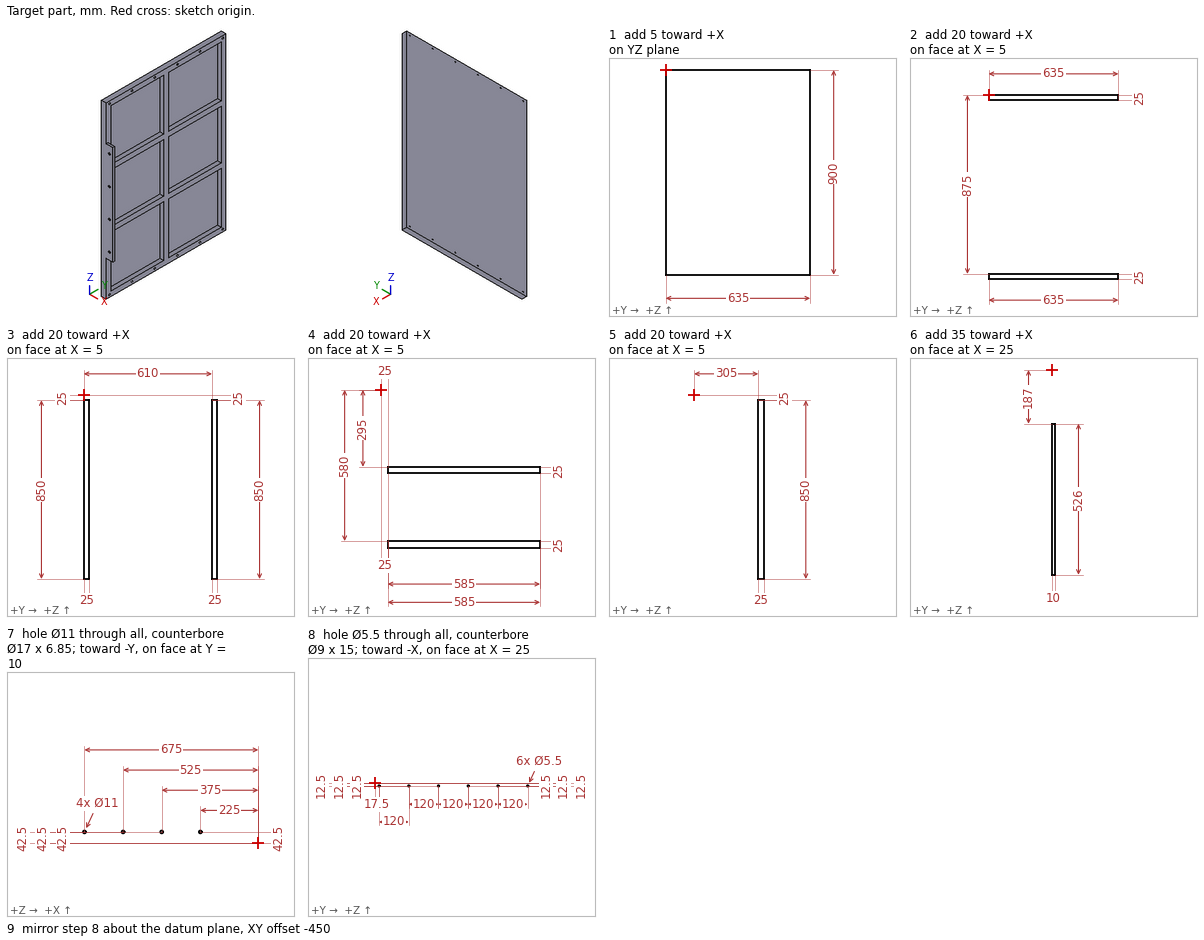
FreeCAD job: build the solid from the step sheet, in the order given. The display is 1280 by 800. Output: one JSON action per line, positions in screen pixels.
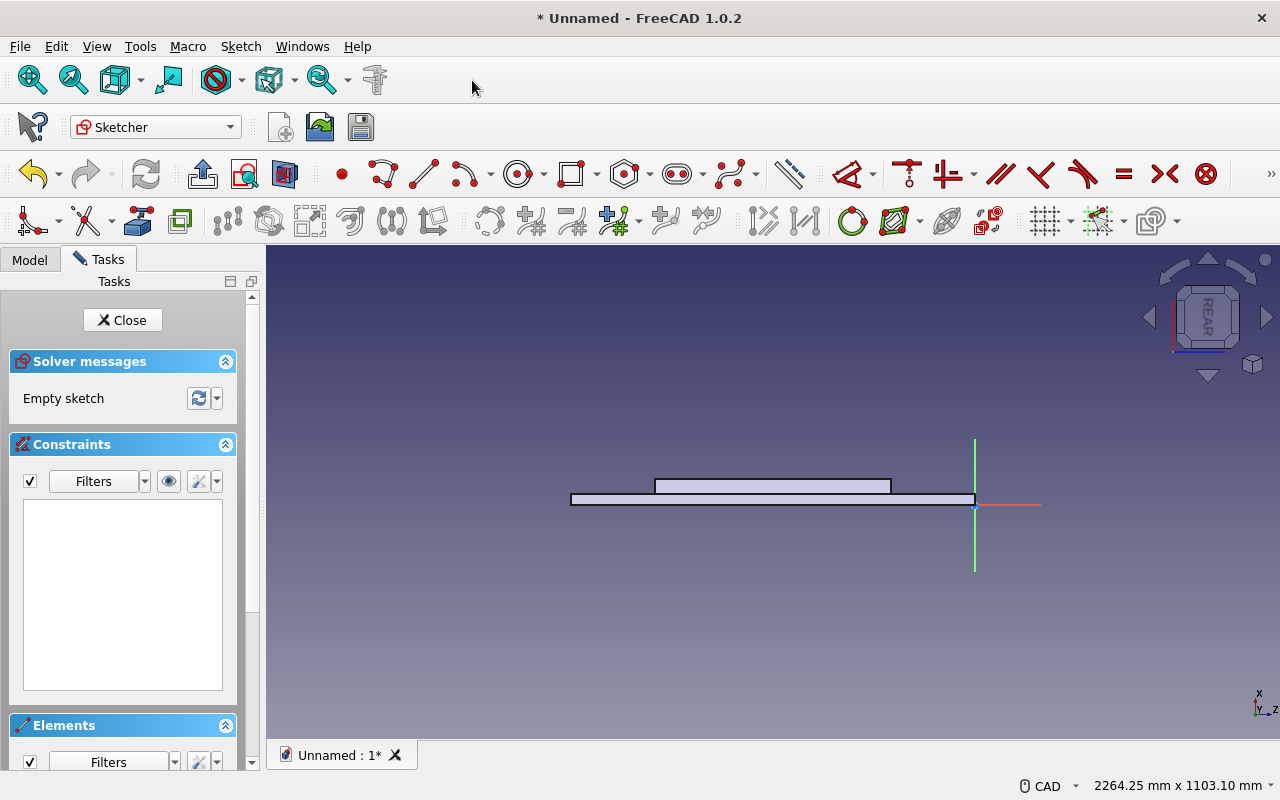
{"action": "scroll", "coordinate": [965, 498], "scroll_direction": "up", "scroll_amount": 3}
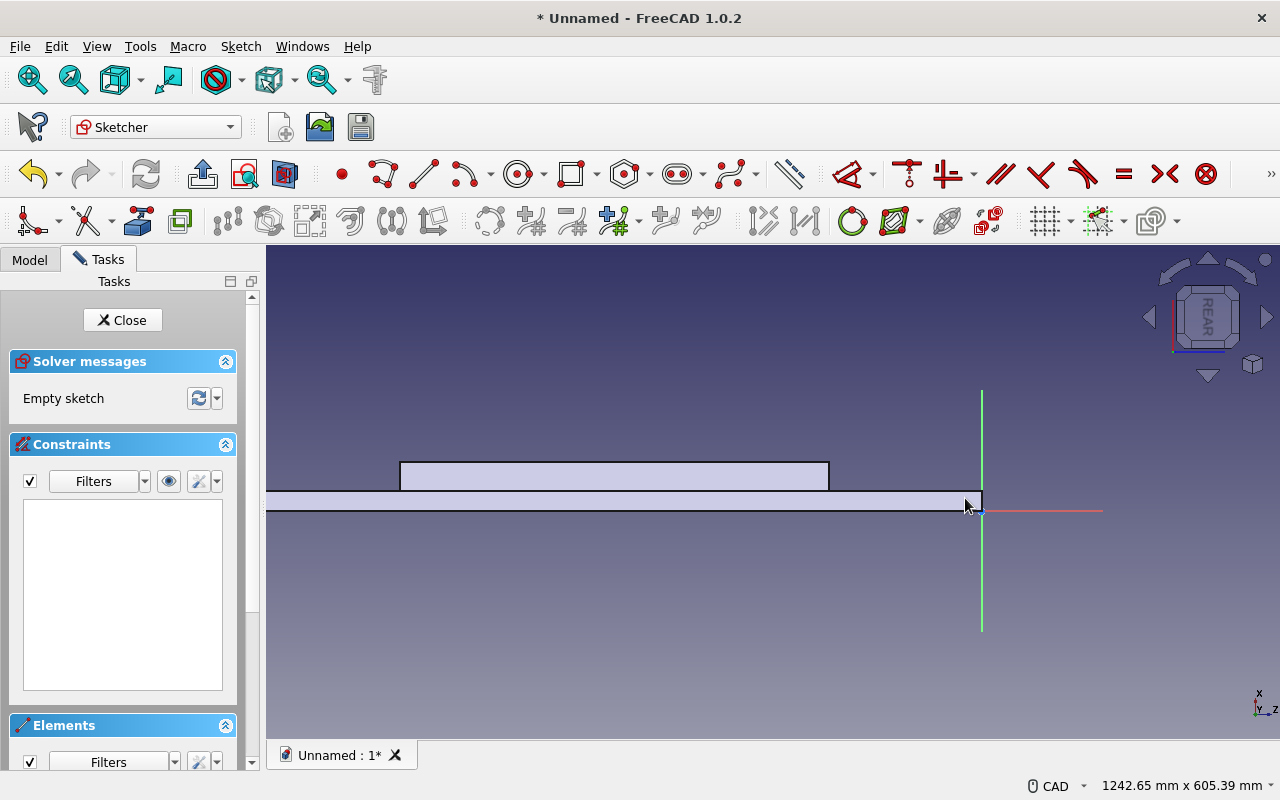
{"action": "left_click", "coordinate": [518, 174]}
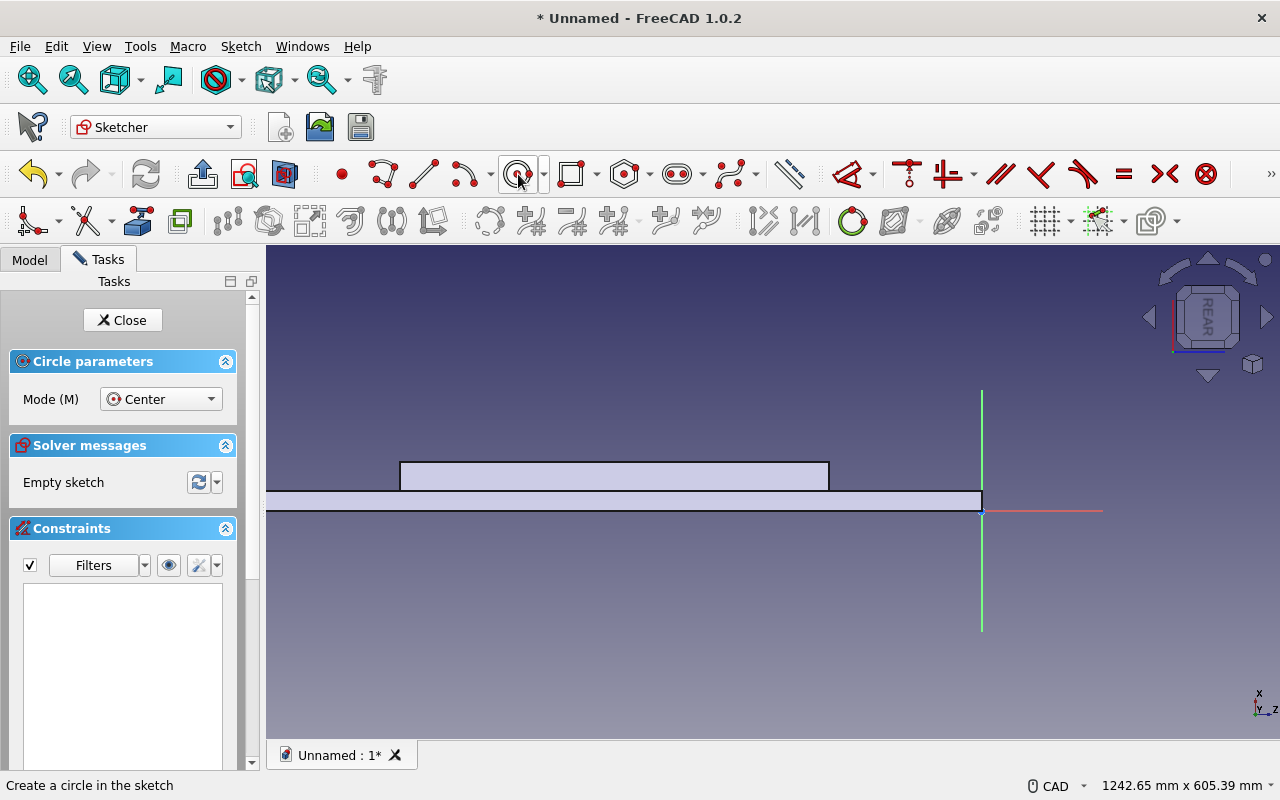
{"action": "scroll", "coordinate": [431, 476], "scroll_direction": "up", "scroll_amount": 9}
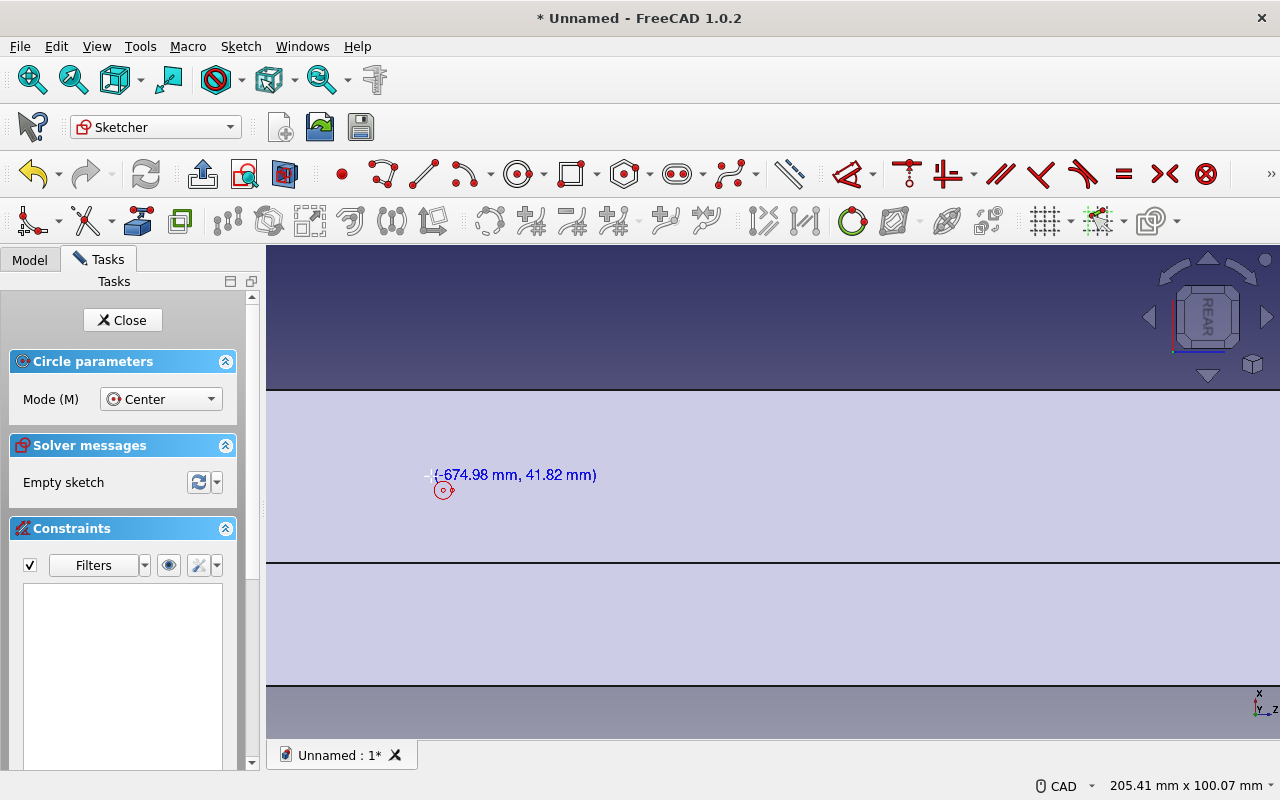
{"action": "scroll", "coordinate": [432, 477], "scroll_direction": "down", "scroll_amount": 9}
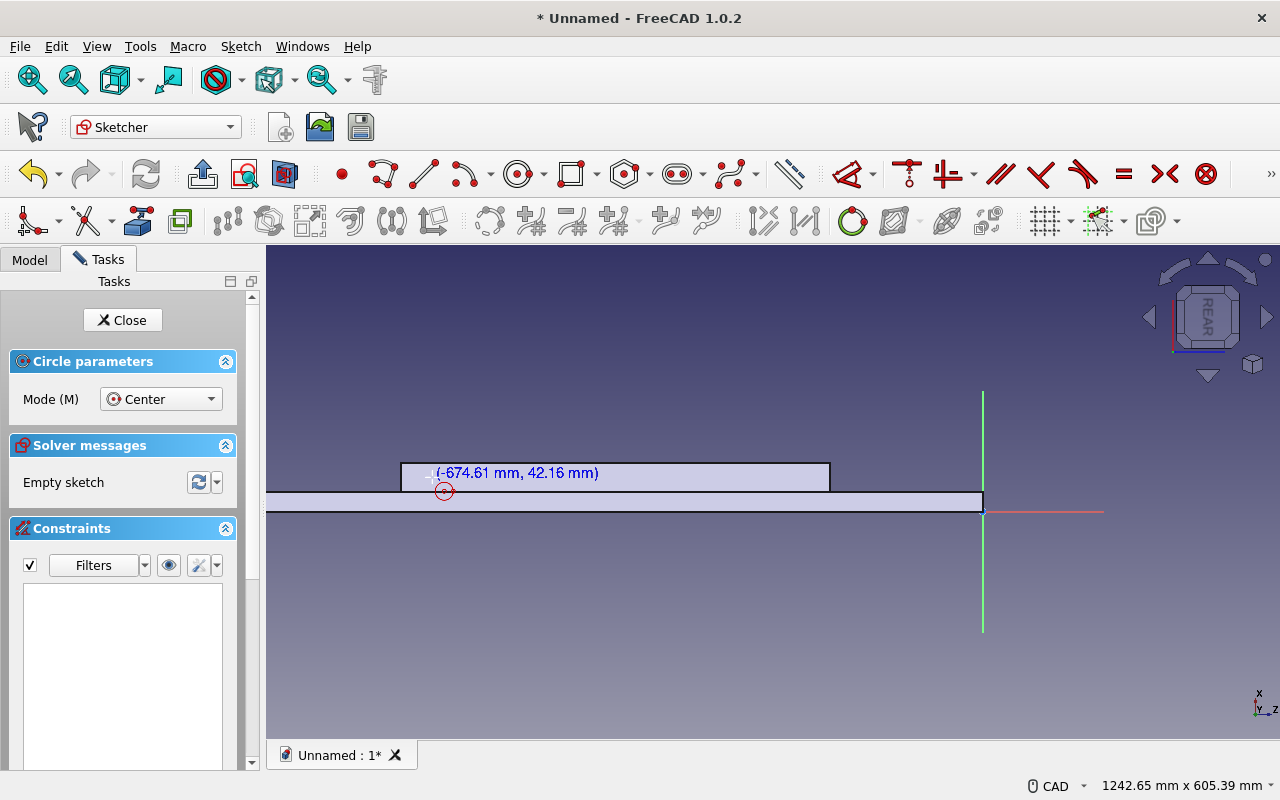
{"action": "left_click", "coordinate": [432, 477]}
{"action": "mouse_move", "coordinate": [435, 474]}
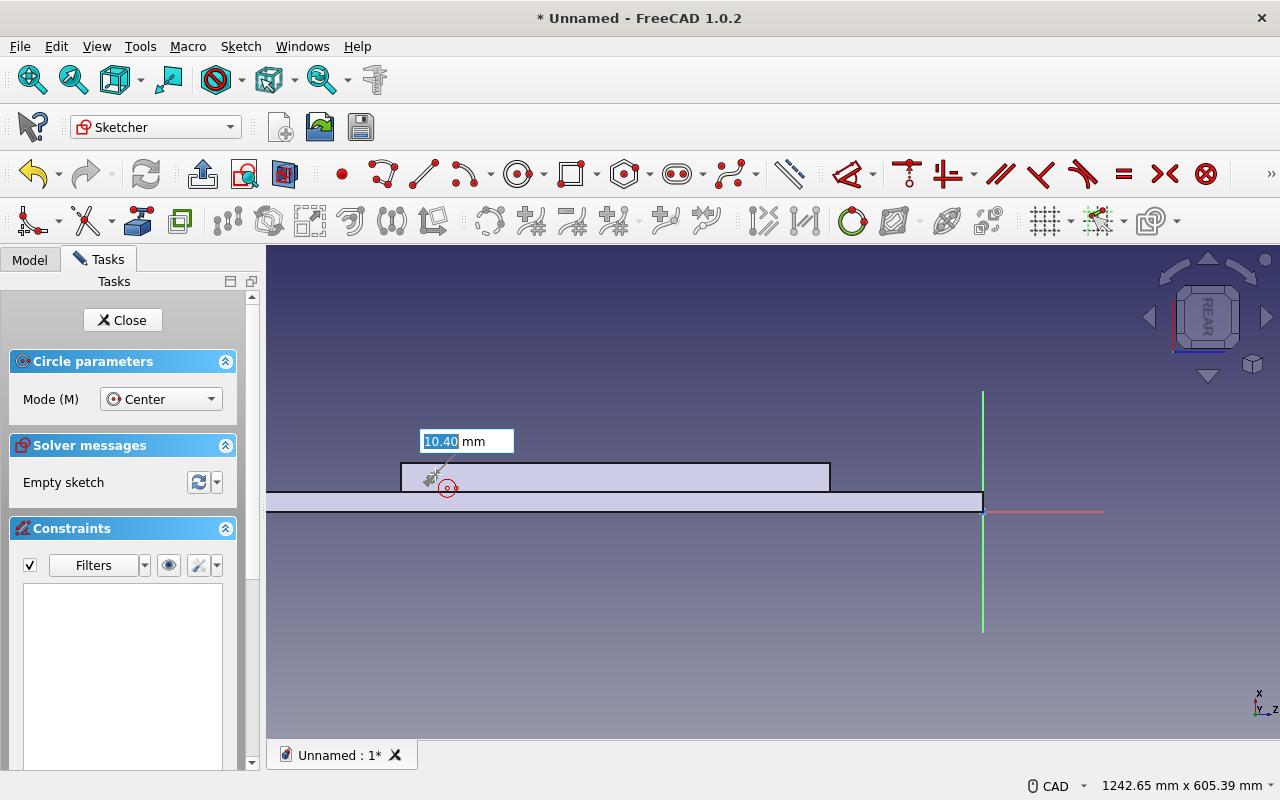
{"action": "type", "text": "11"}
{"action": "key", "text": "Return"}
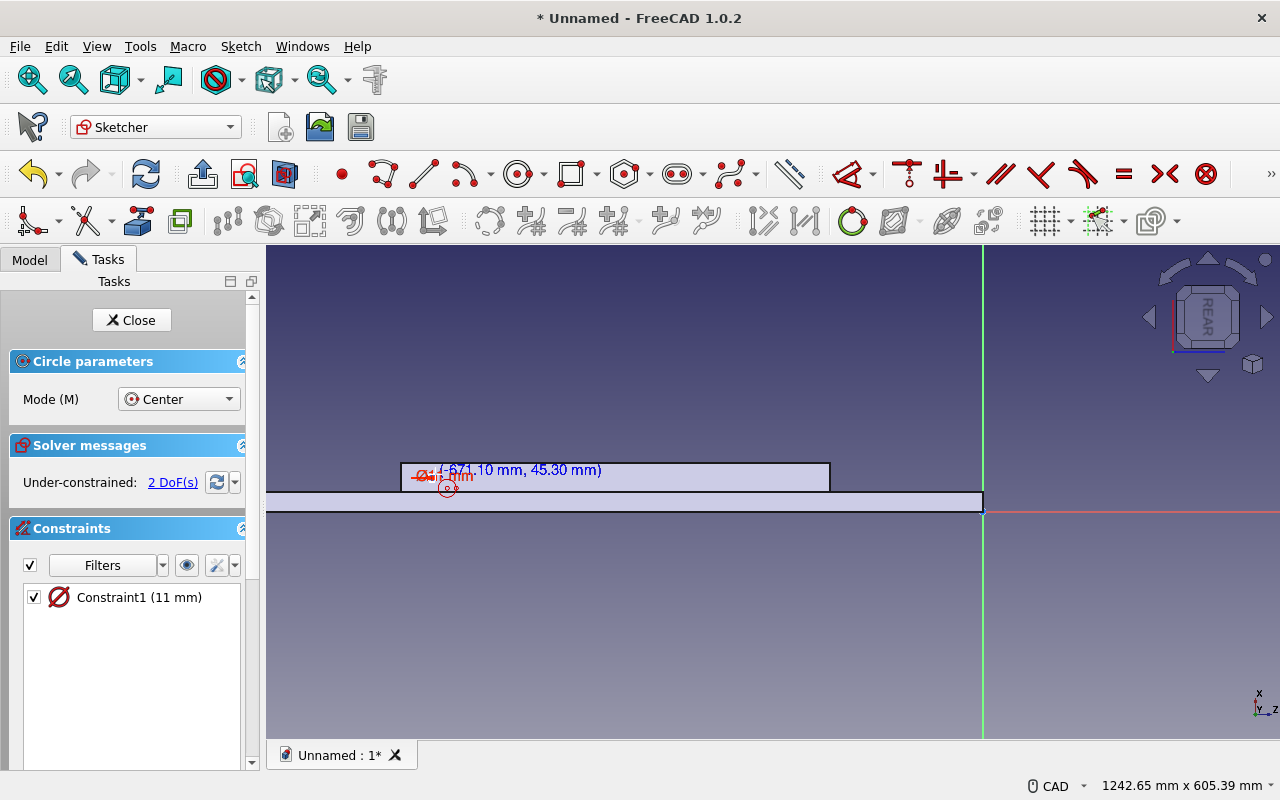
{"action": "scroll", "coordinate": [554, 477], "scroll_direction": "up", "scroll_amount": 9}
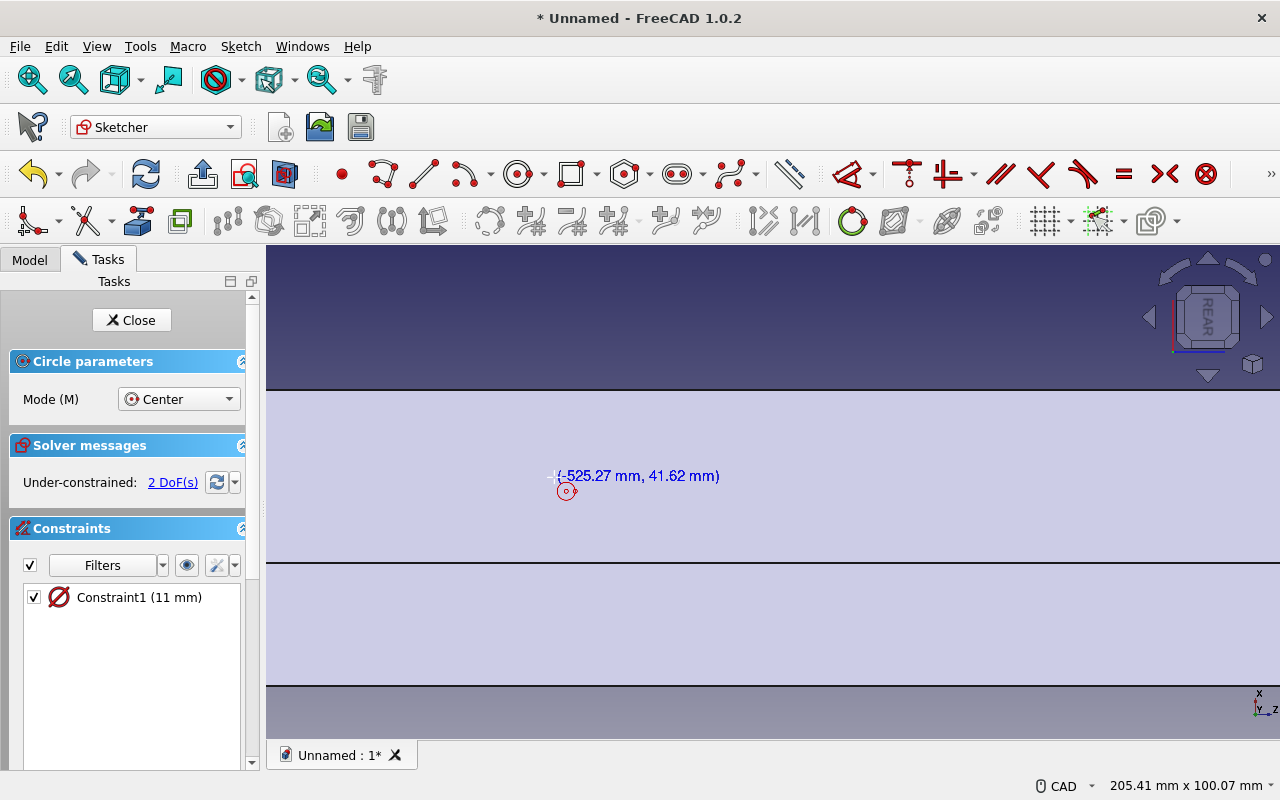
{"action": "scroll", "coordinate": [554, 477], "scroll_direction": "down", "scroll_amount": 9}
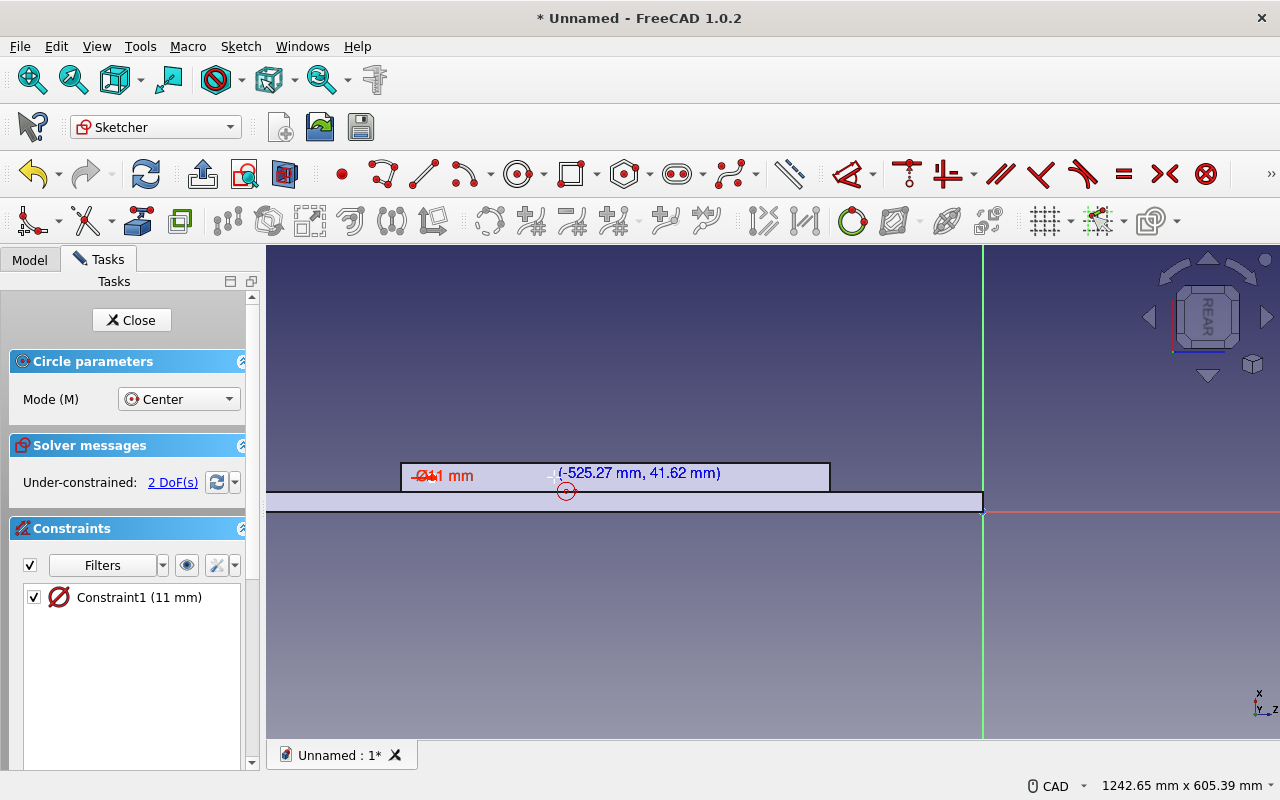
{"action": "left_click", "coordinate": [554, 477]}
{"action": "mouse_move", "coordinate": [557, 474]}